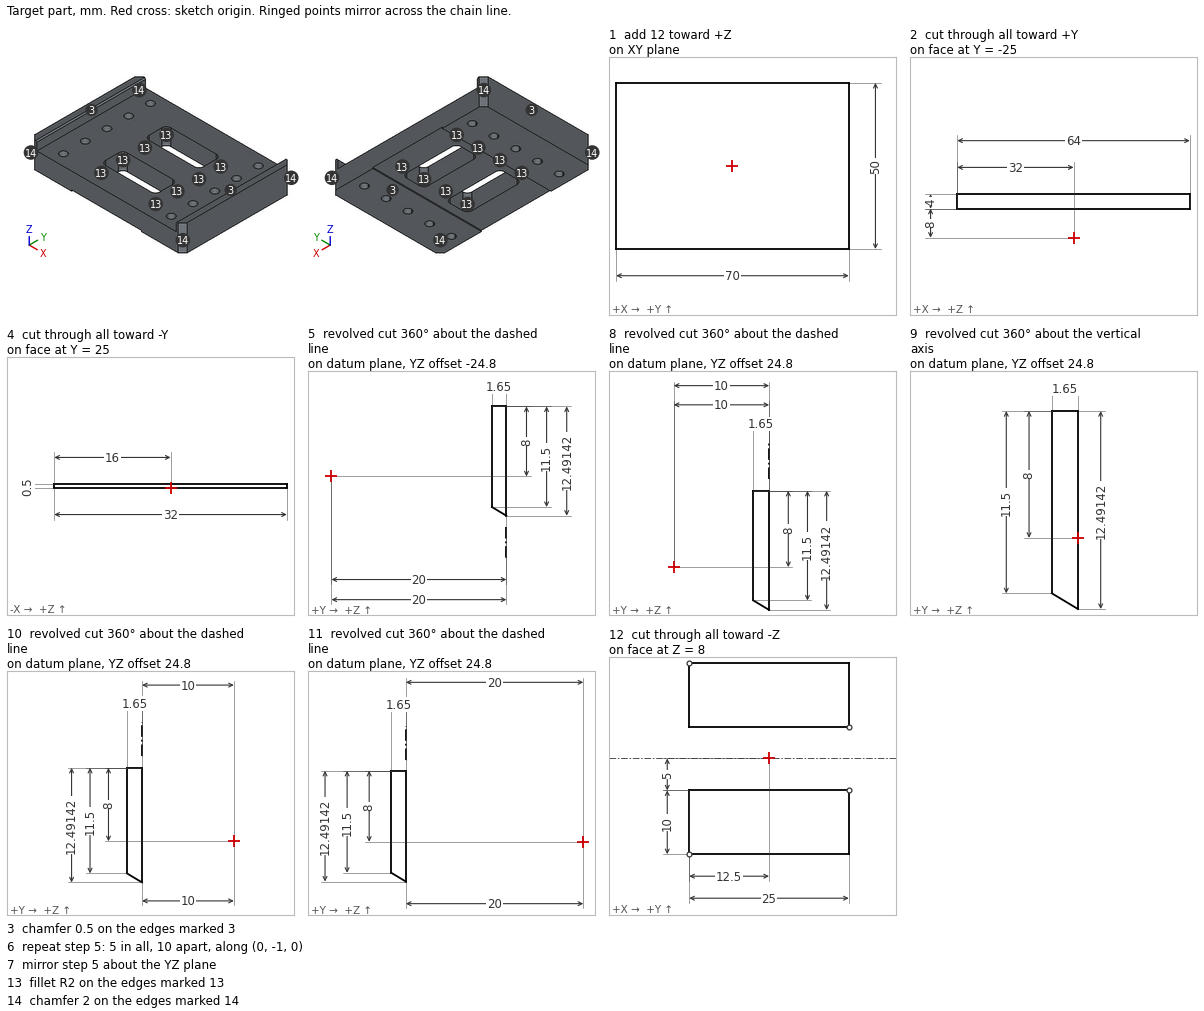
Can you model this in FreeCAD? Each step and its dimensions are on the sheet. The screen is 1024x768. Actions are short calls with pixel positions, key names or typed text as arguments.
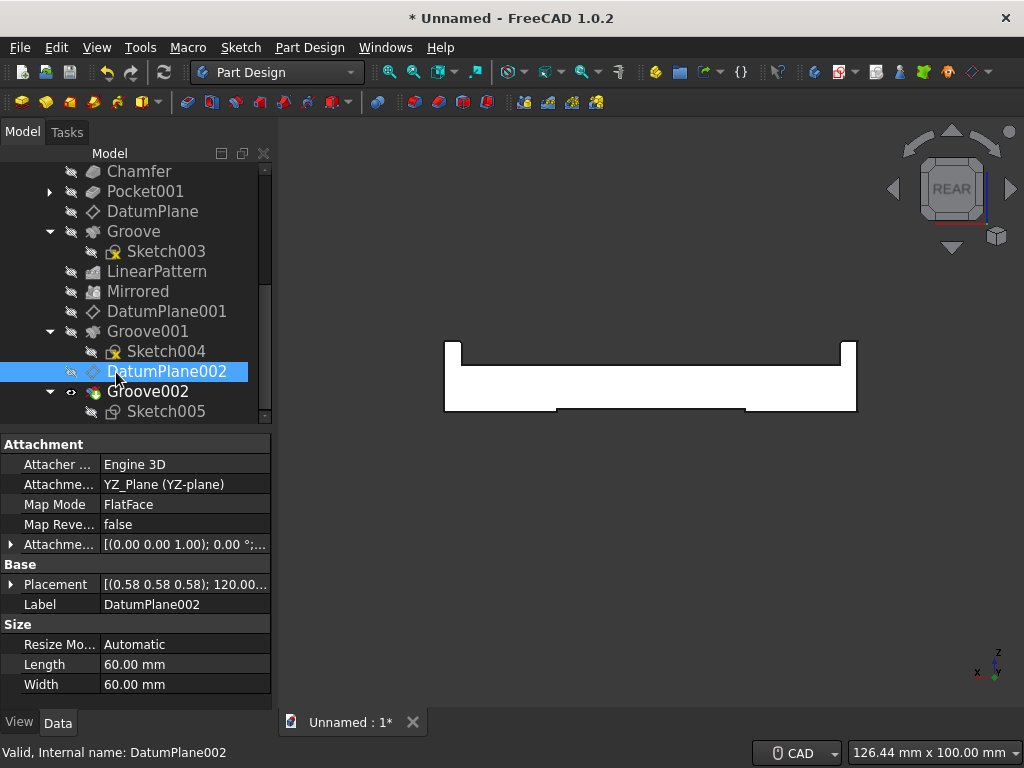
scroll(140, 287, down, 3)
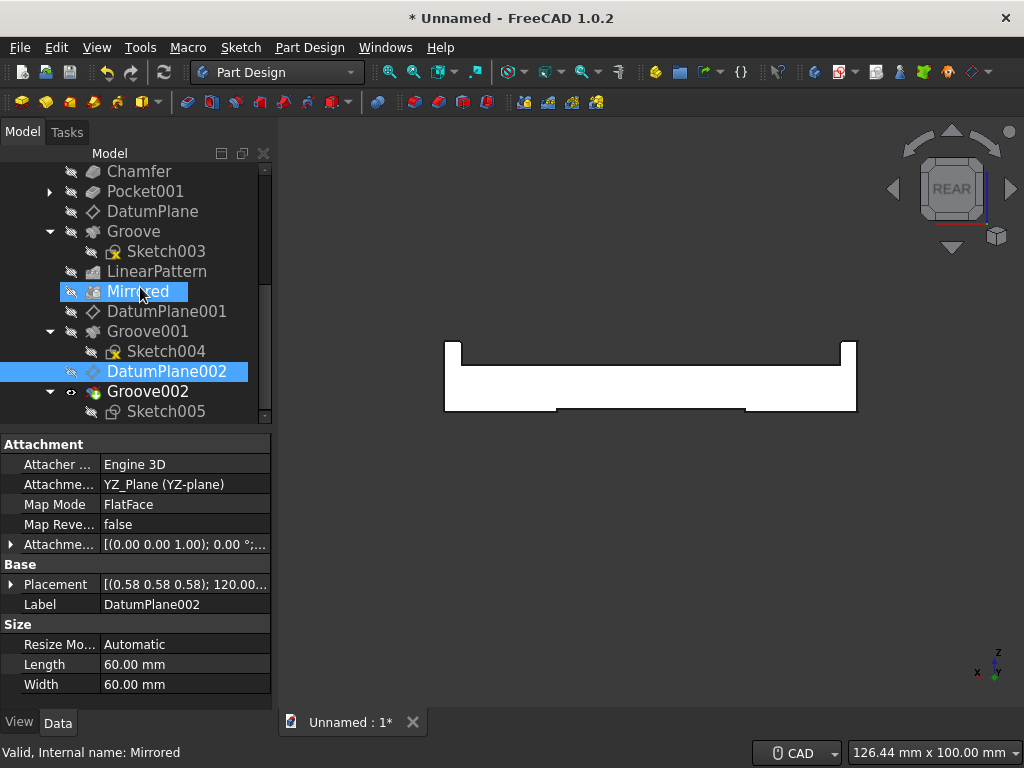
scroll(140, 287, up, 15)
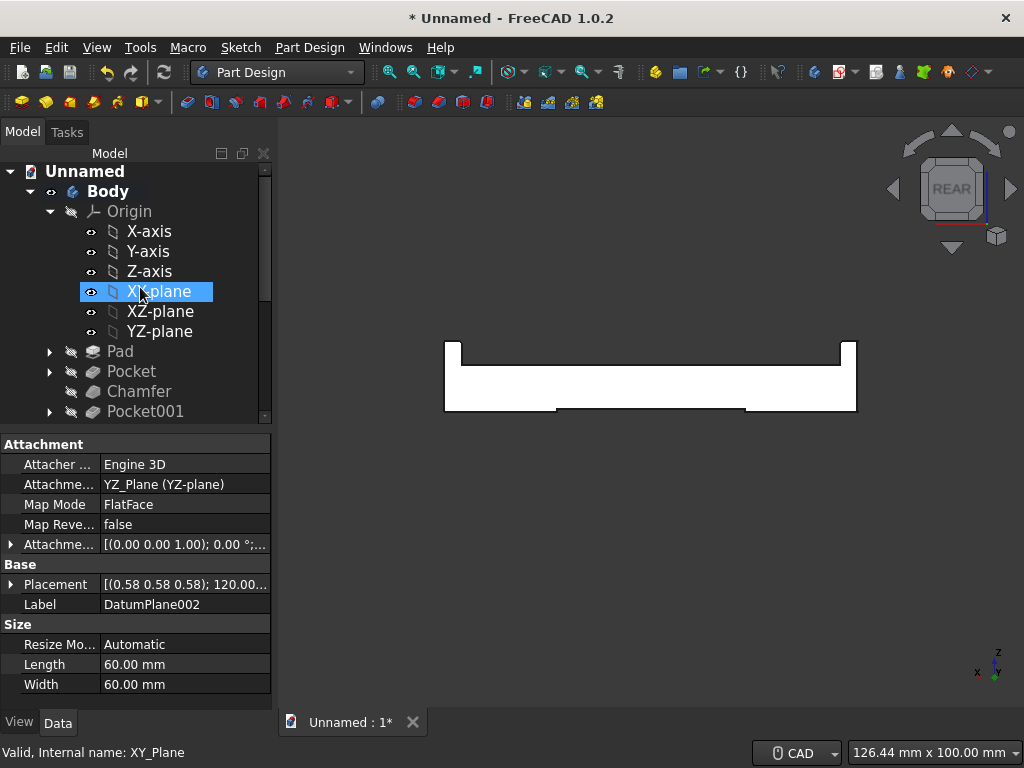
click(136, 332)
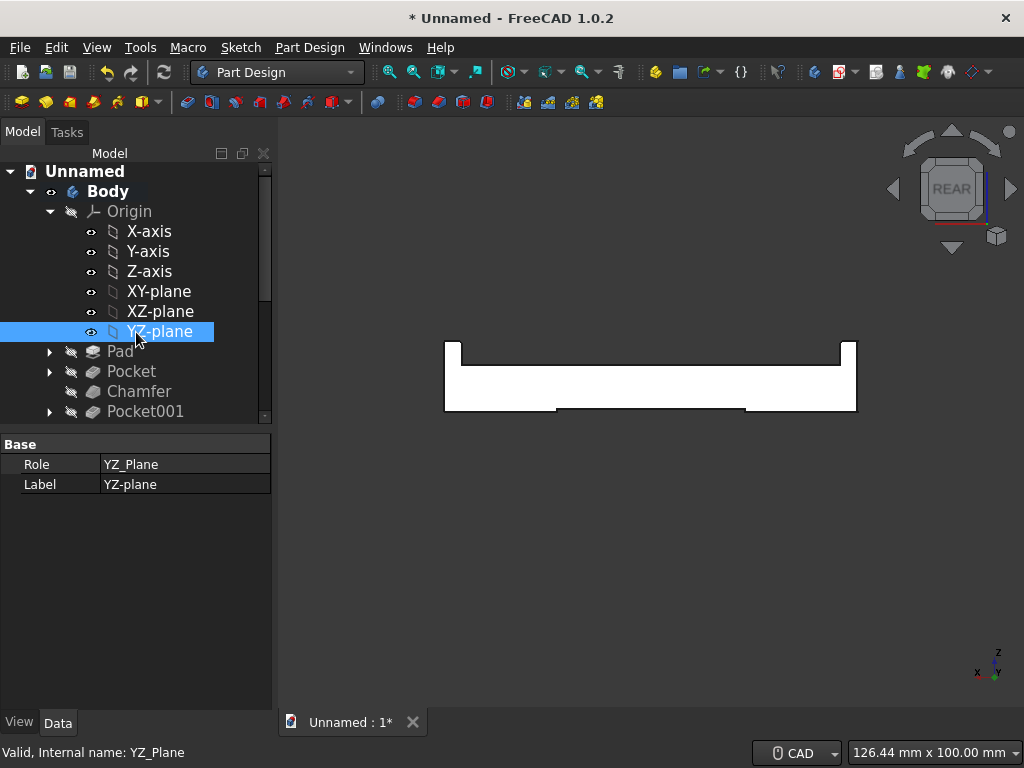
click(972, 72)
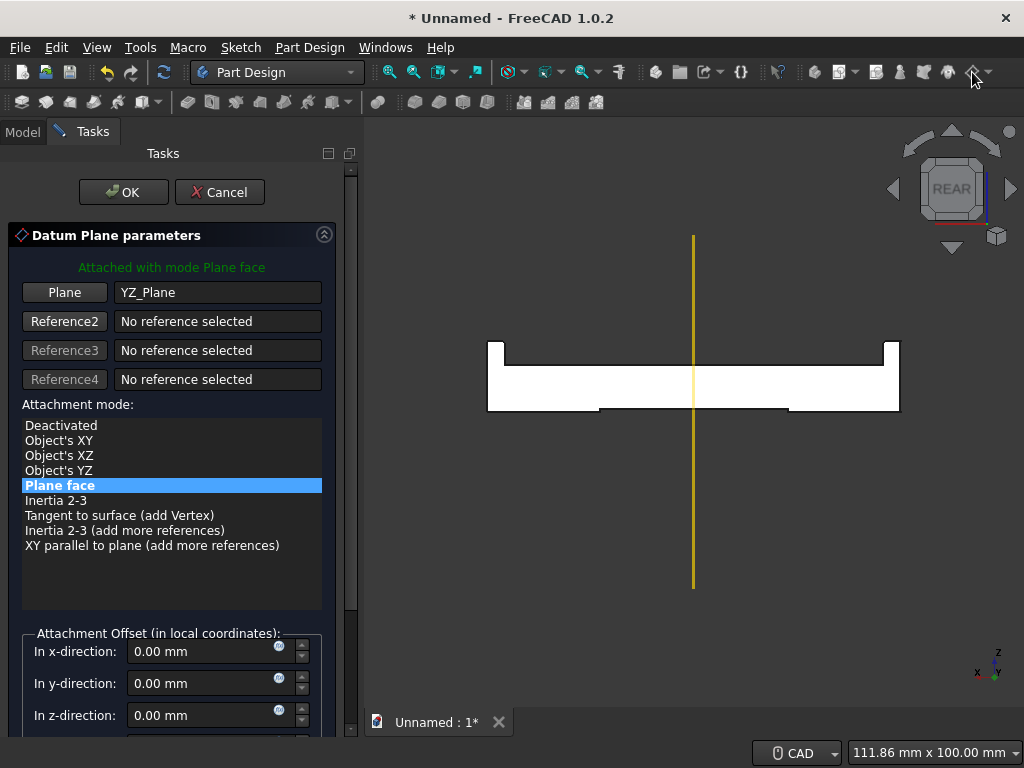
triple_click(210, 715)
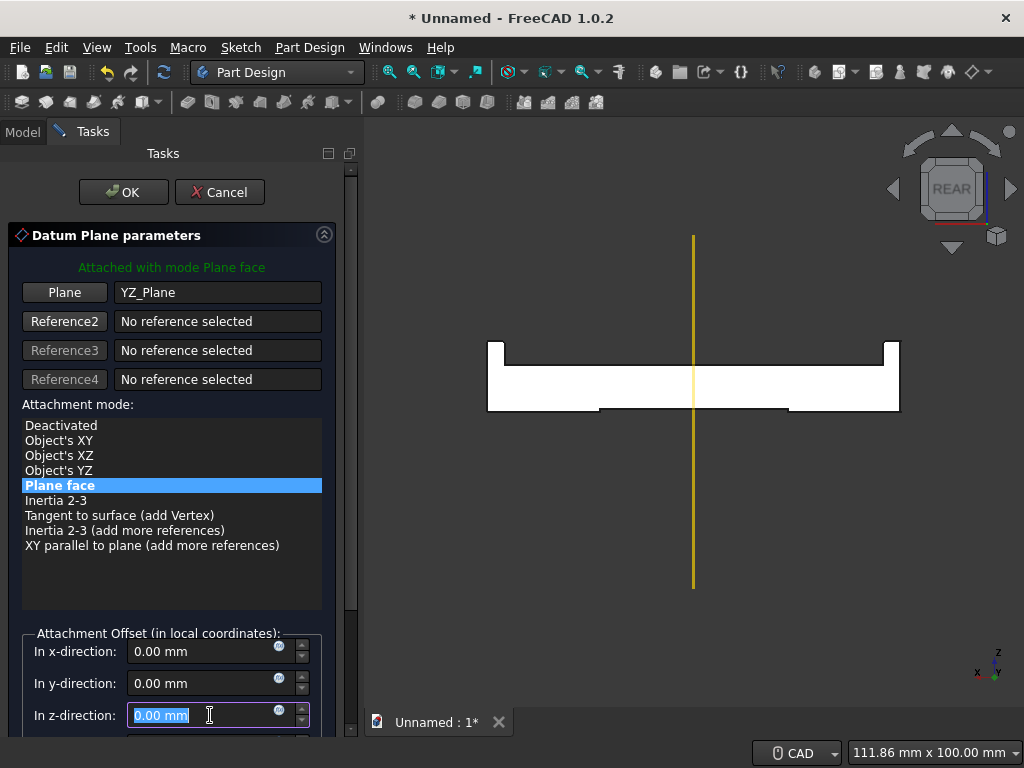
text(24.8)
key(Tab)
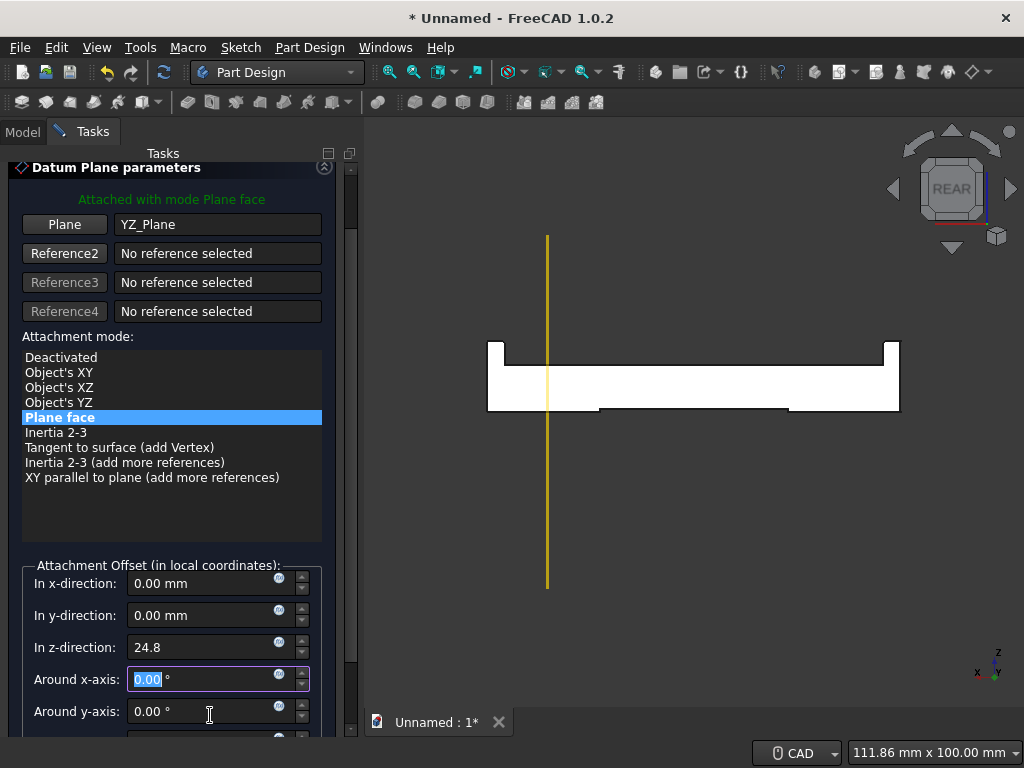
scroll(351, 450, up, 2)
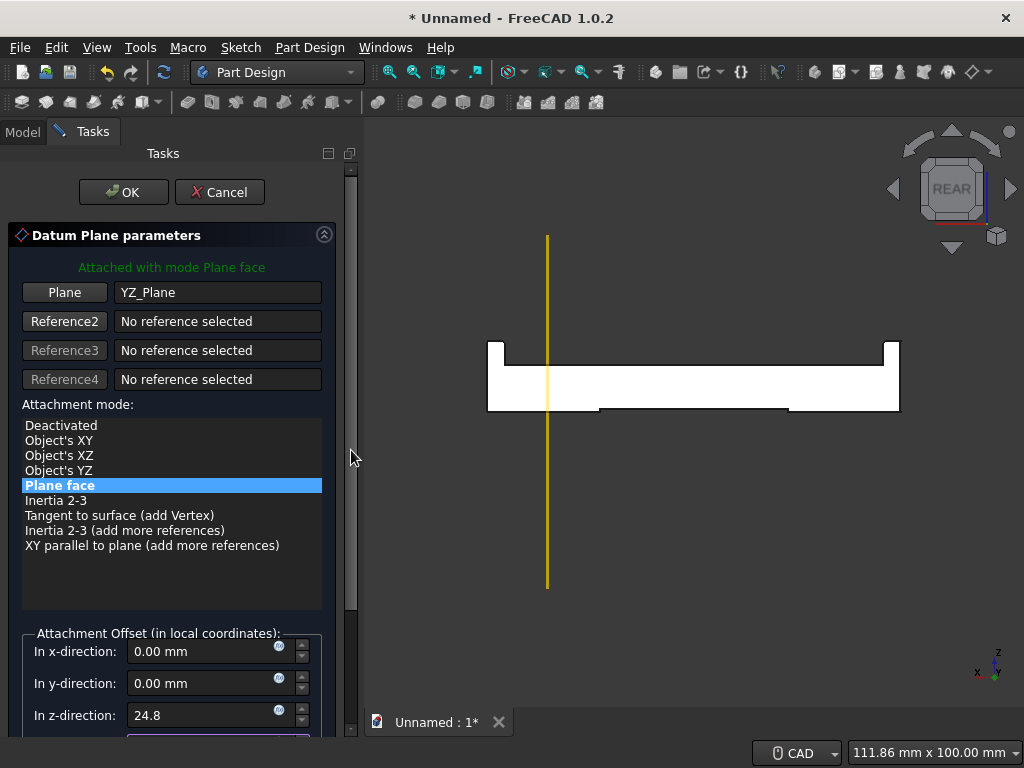
click(124, 192)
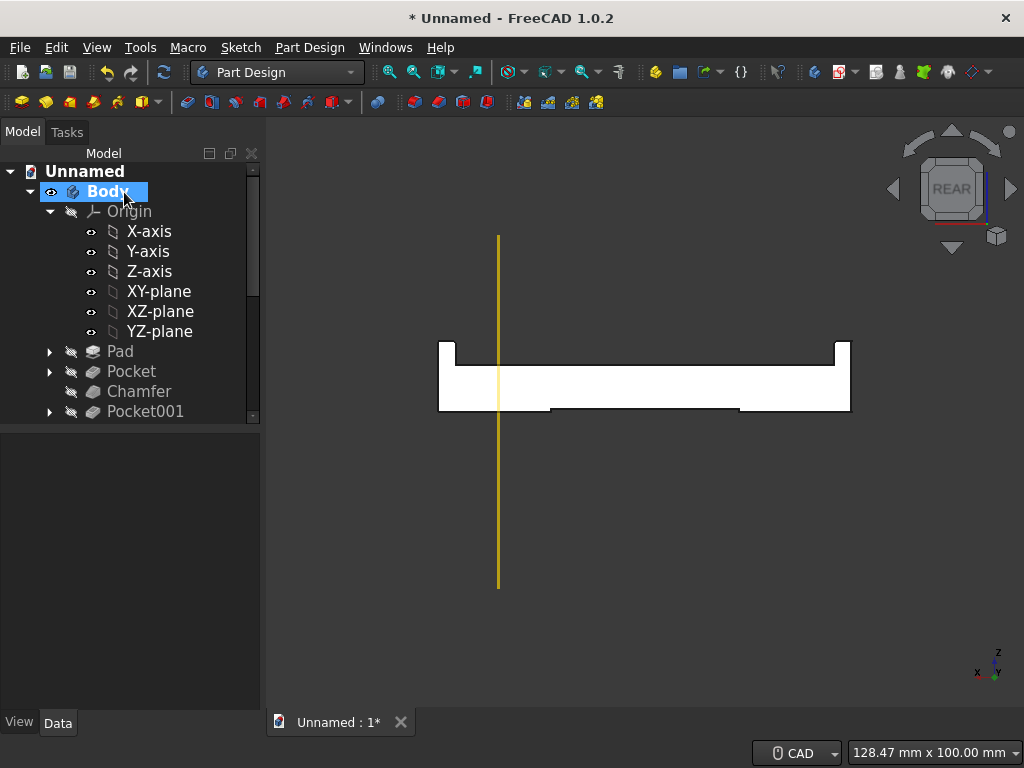
scroll(100, 287, down, 3)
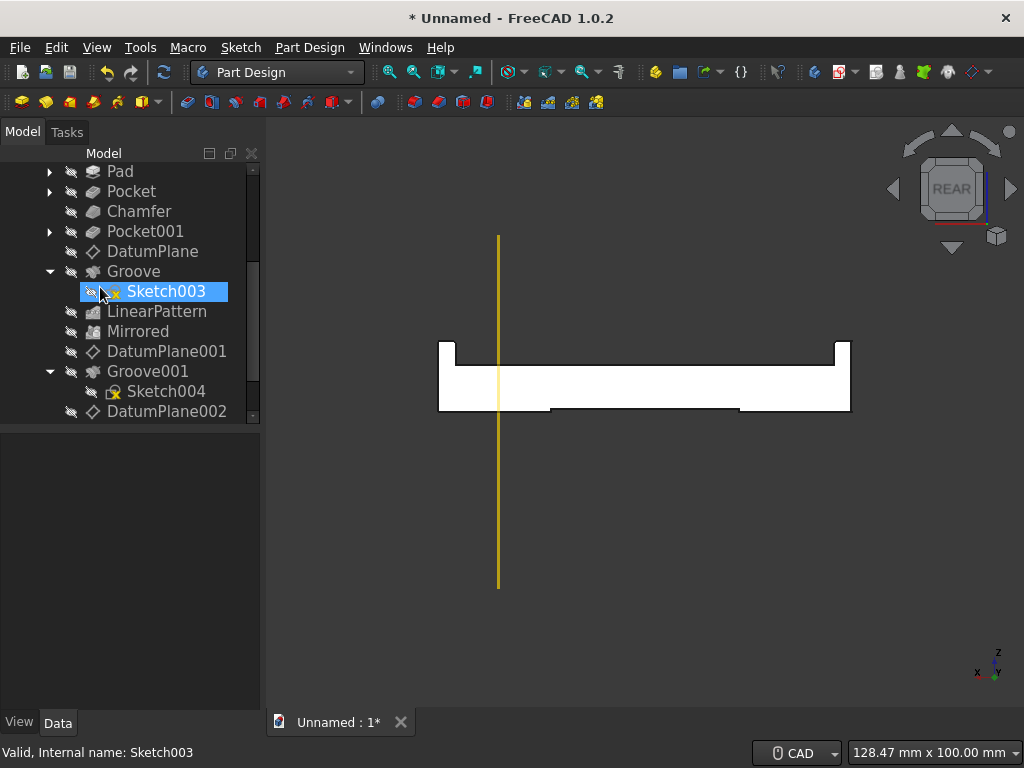
scroll(140, 287, up, 15)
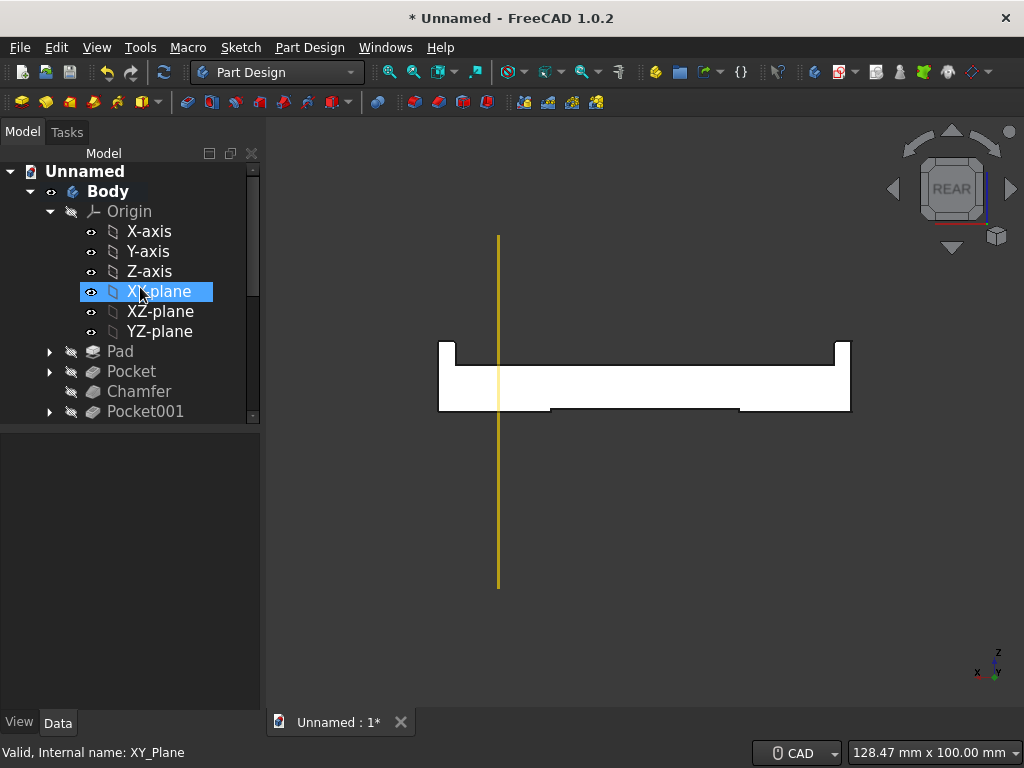
scroll(100, 287, down, 6)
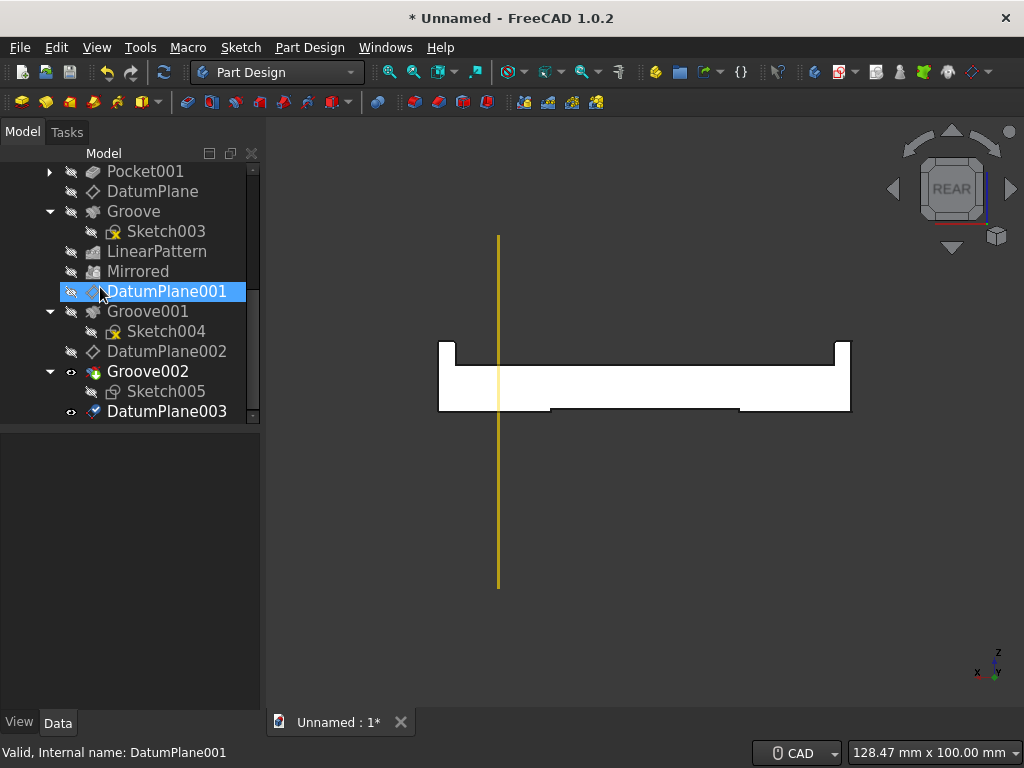
click(116, 412)